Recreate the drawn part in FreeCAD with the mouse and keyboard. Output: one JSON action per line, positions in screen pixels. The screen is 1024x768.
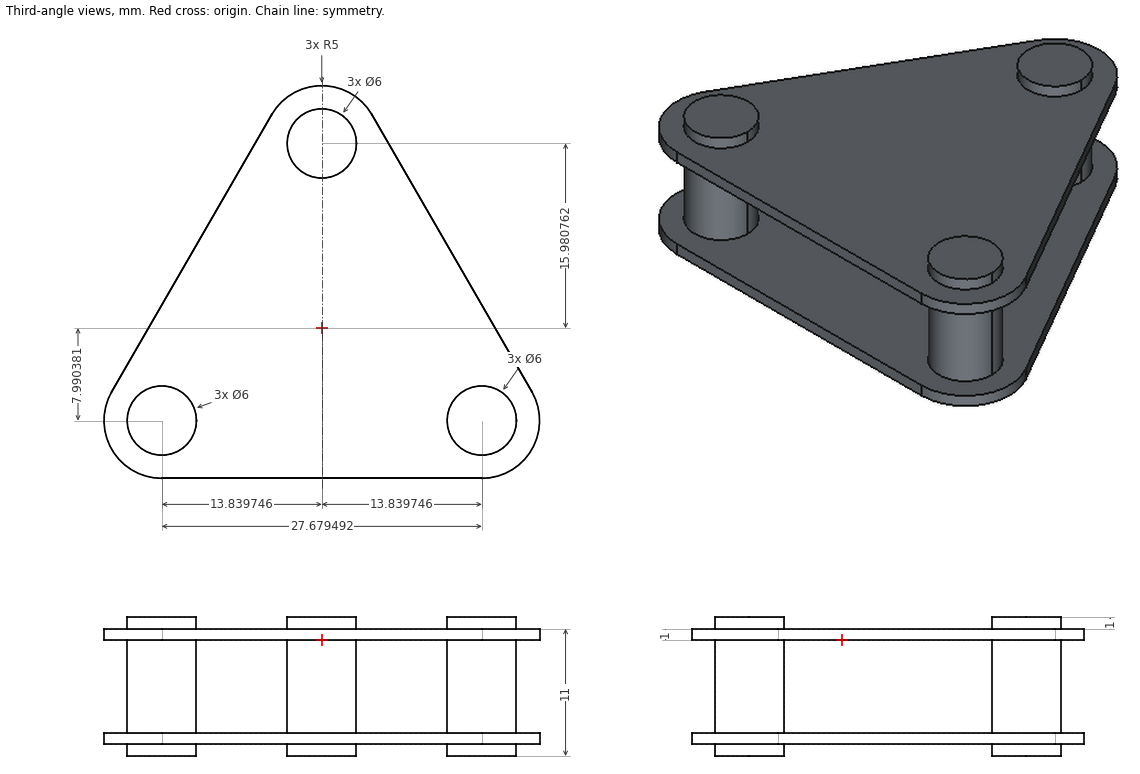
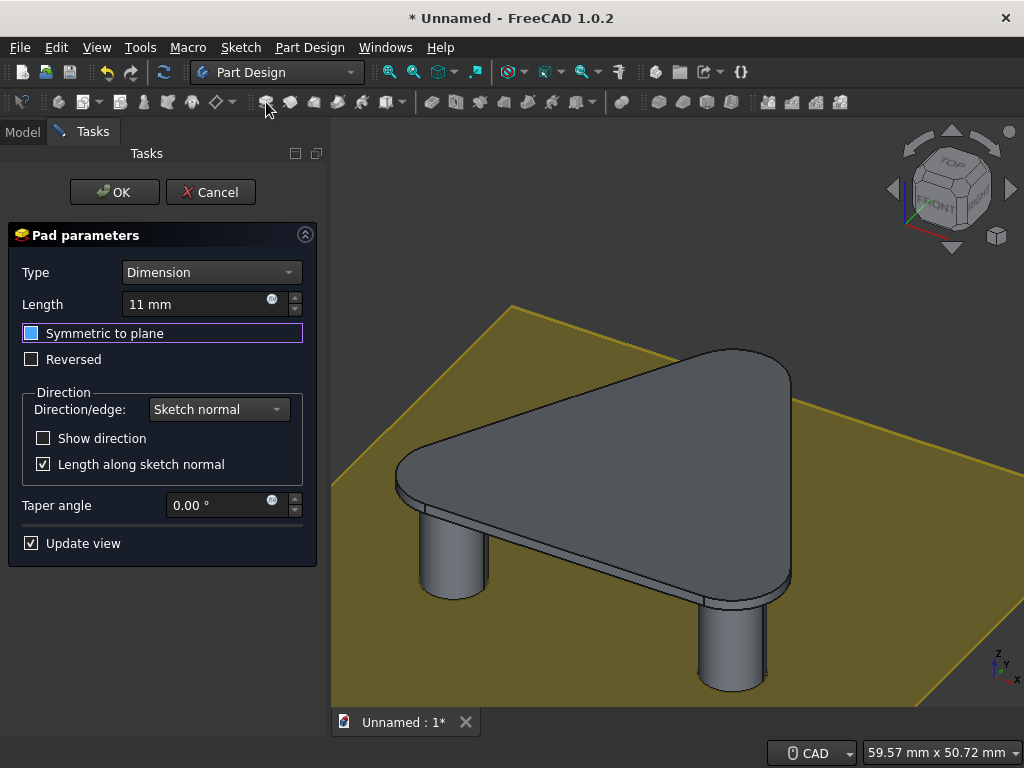
{"action": "left_click", "coordinate": [115, 192]}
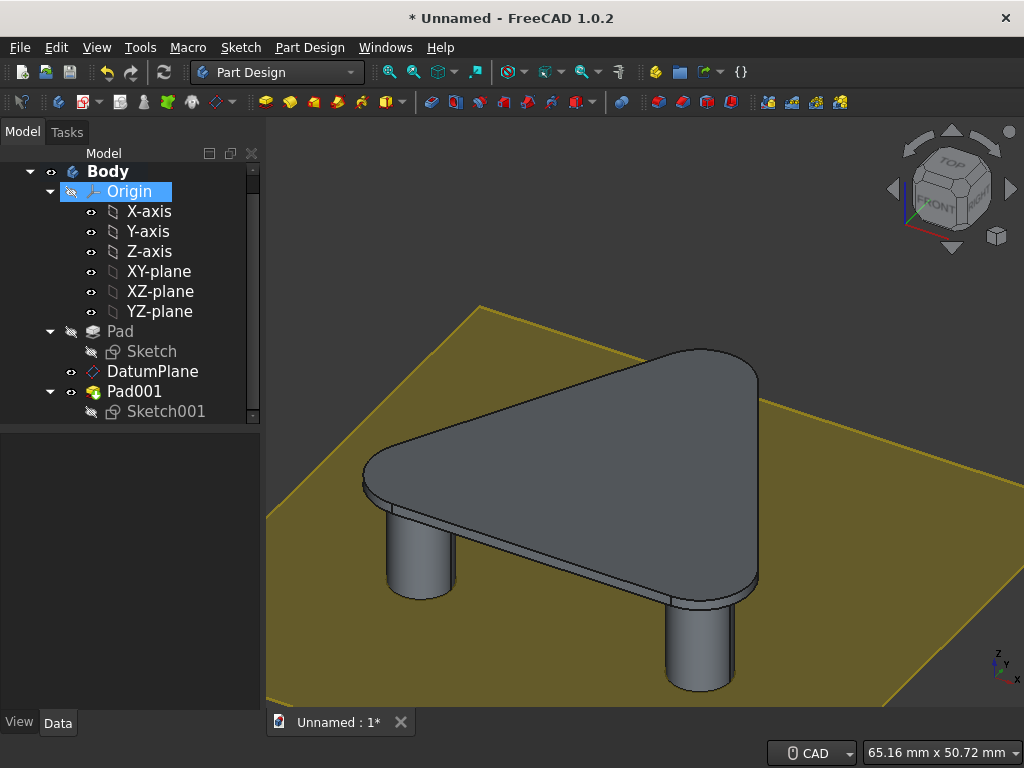
{"action": "left_click", "coordinate": [116, 372]}
{"action": "key", "text": "space"}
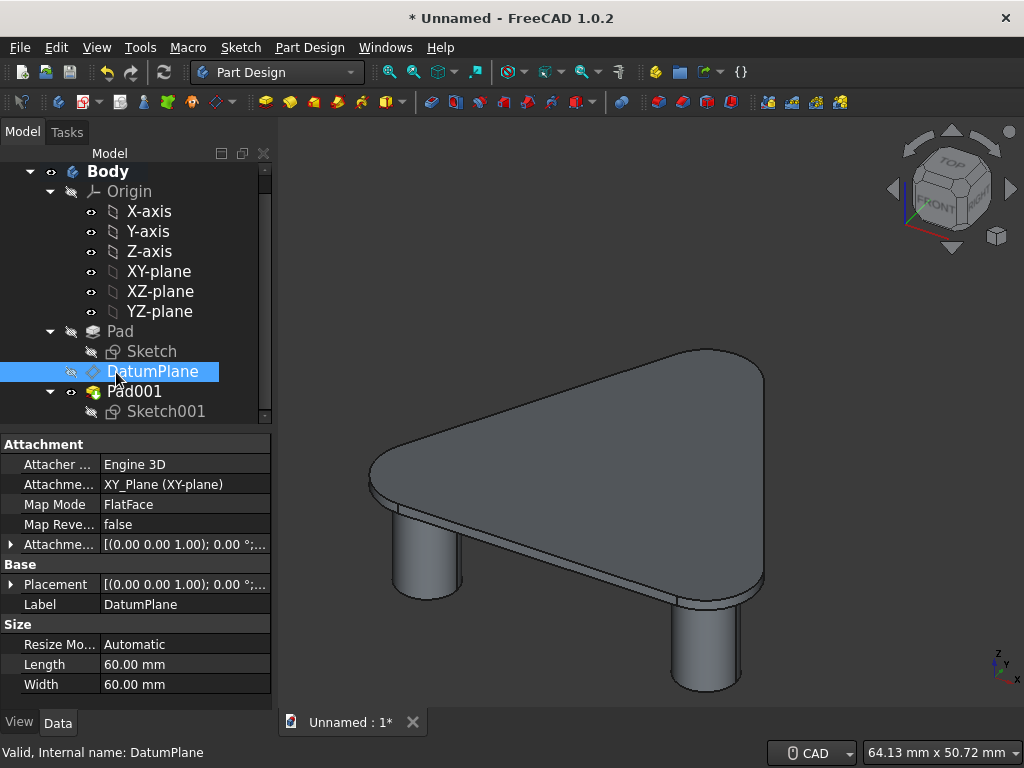
{"action": "left_click", "coordinate": [390, 72]}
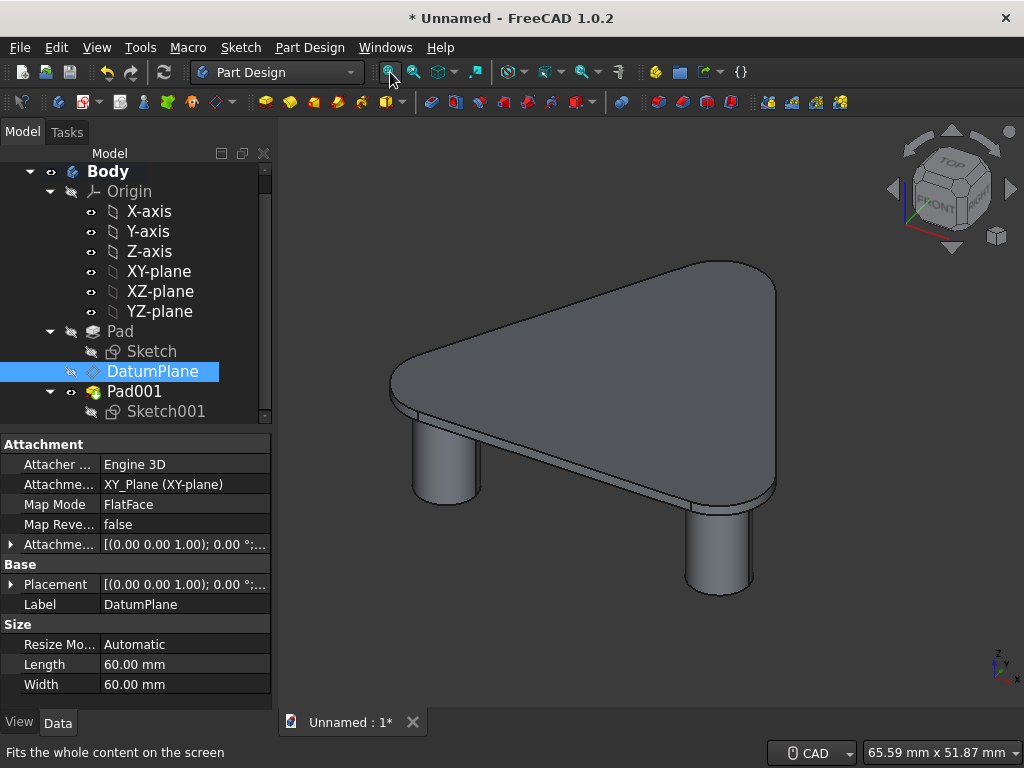
{"action": "left_click", "coordinate": [136, 272]}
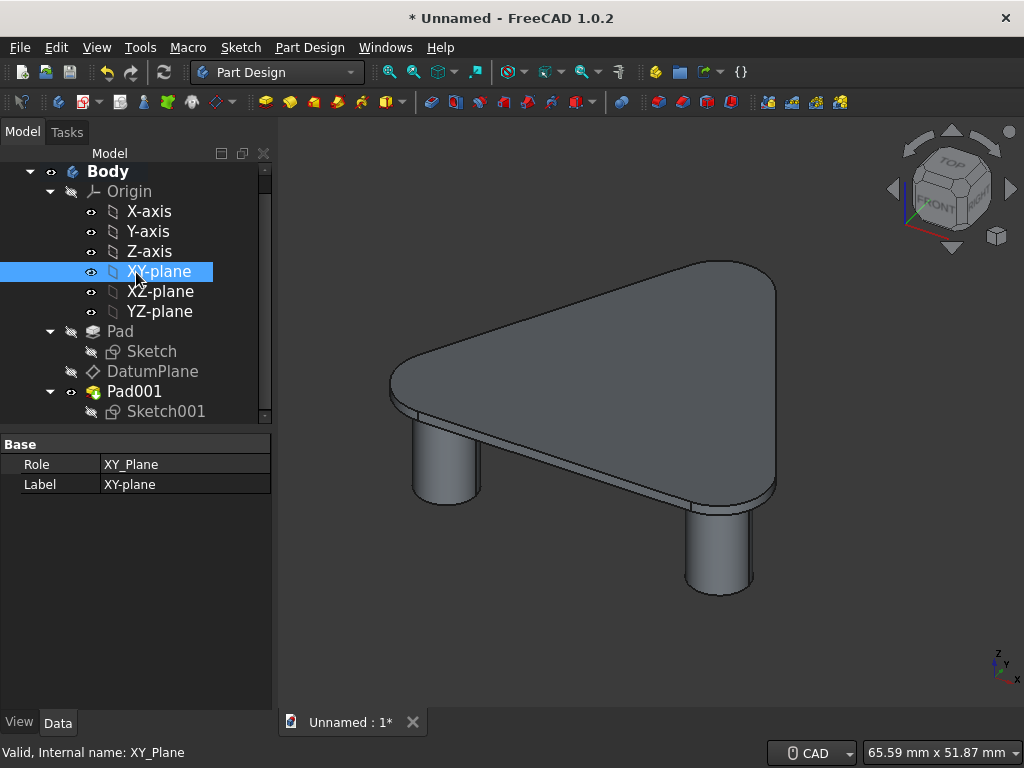
{"action": "left_click", "coordinate": [216, 102]}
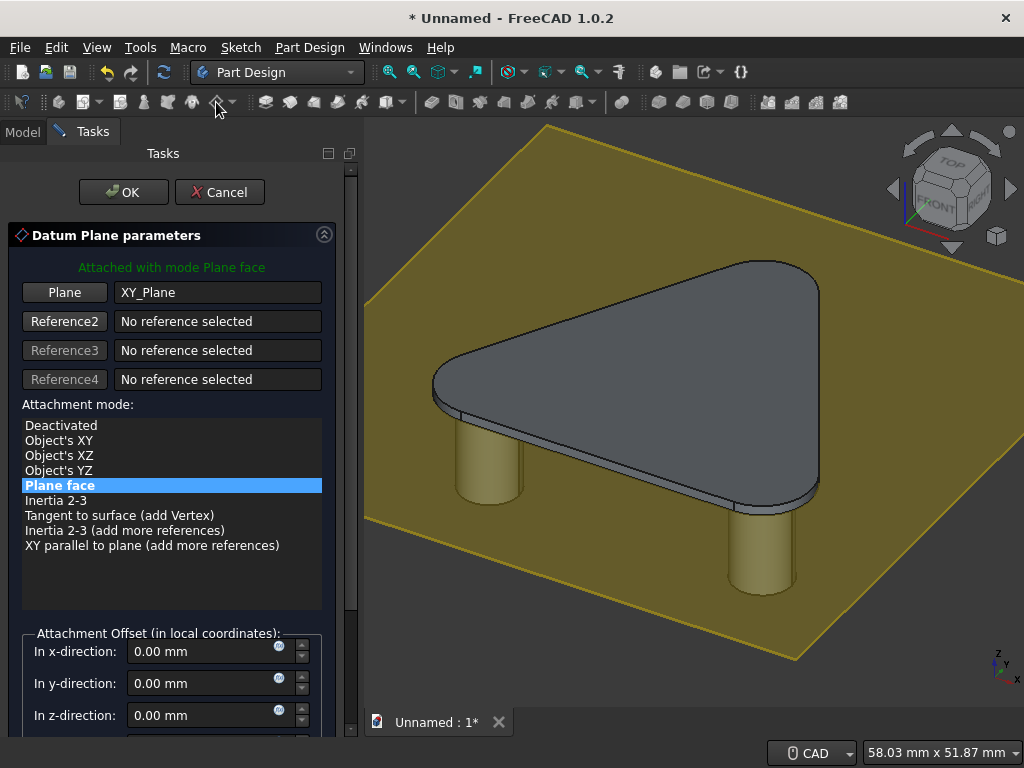
{"action": "triple_click", "coordinate": [210, 715]}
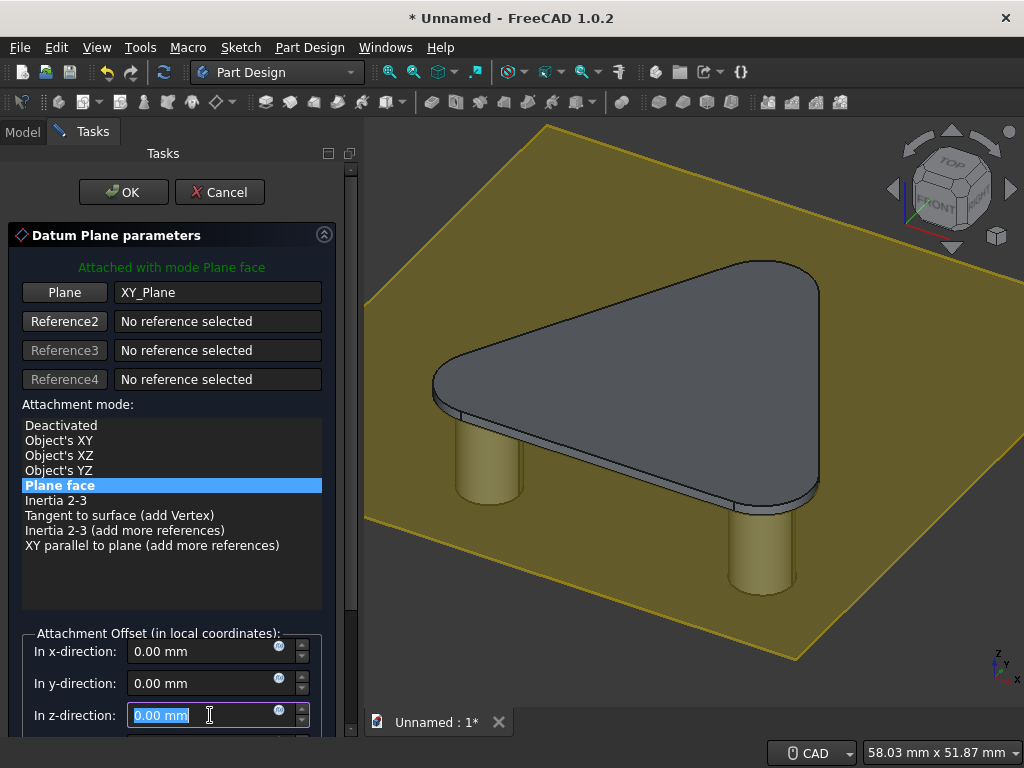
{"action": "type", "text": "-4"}
{"action": "key", "text": "Tab"}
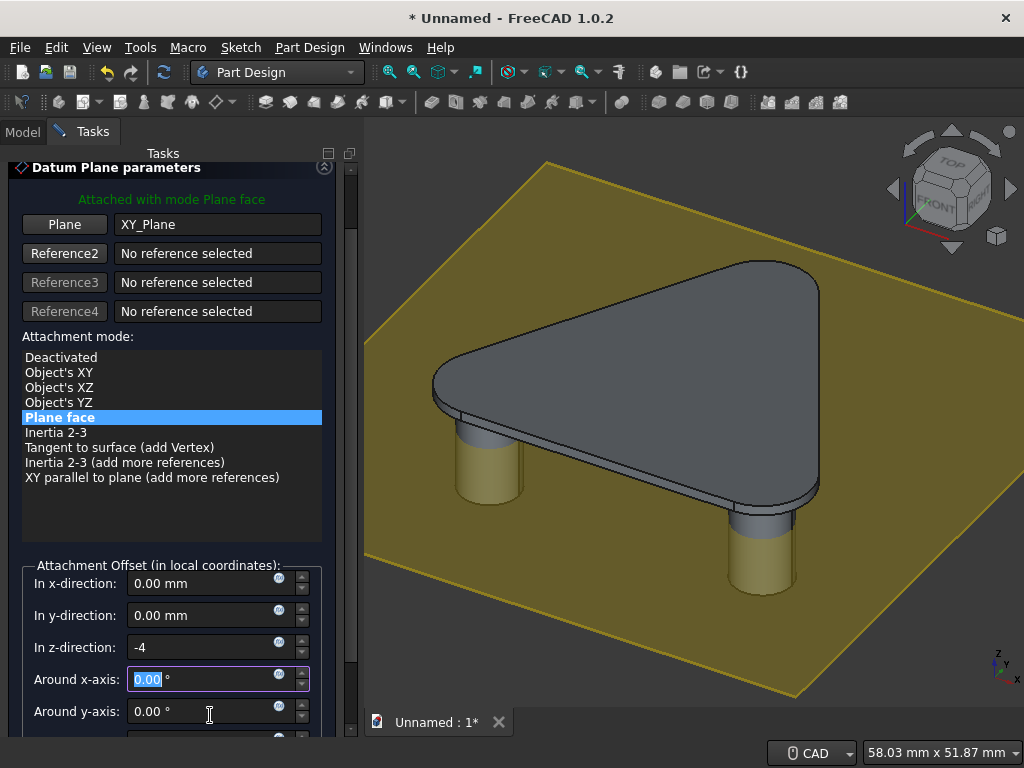
{"action": "scroll", "coordinate": [351, 450], "scroll_direction": "up", "scroll_amount": 2}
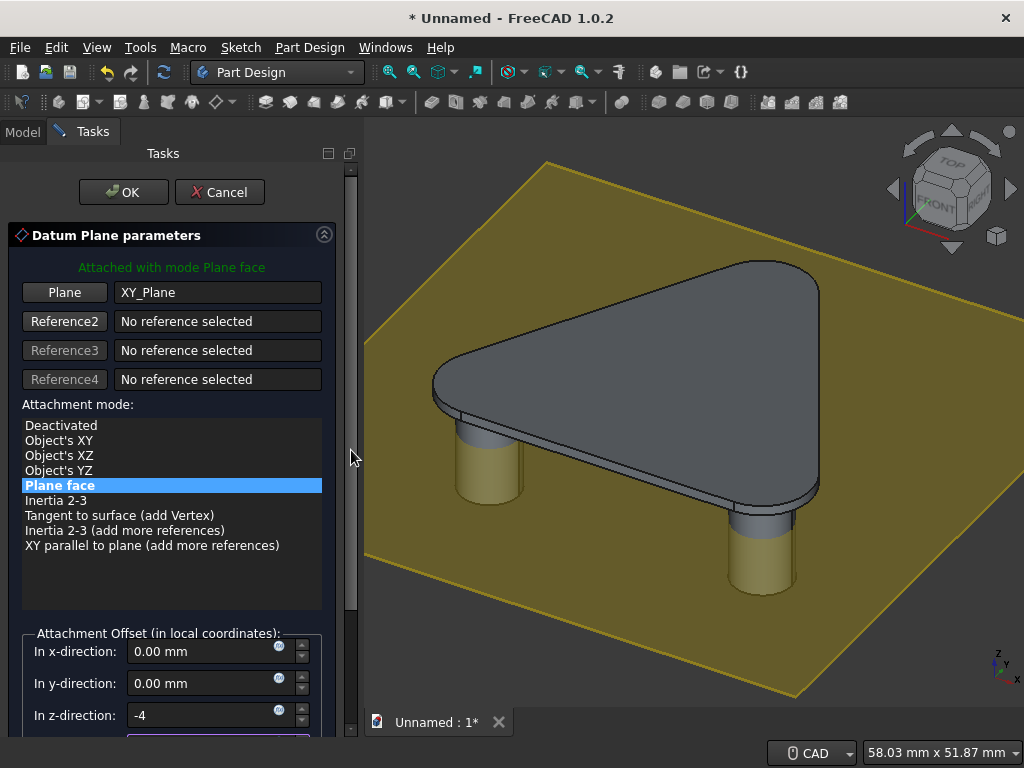
{"action": "left_click", "coordinate": [124, 192]}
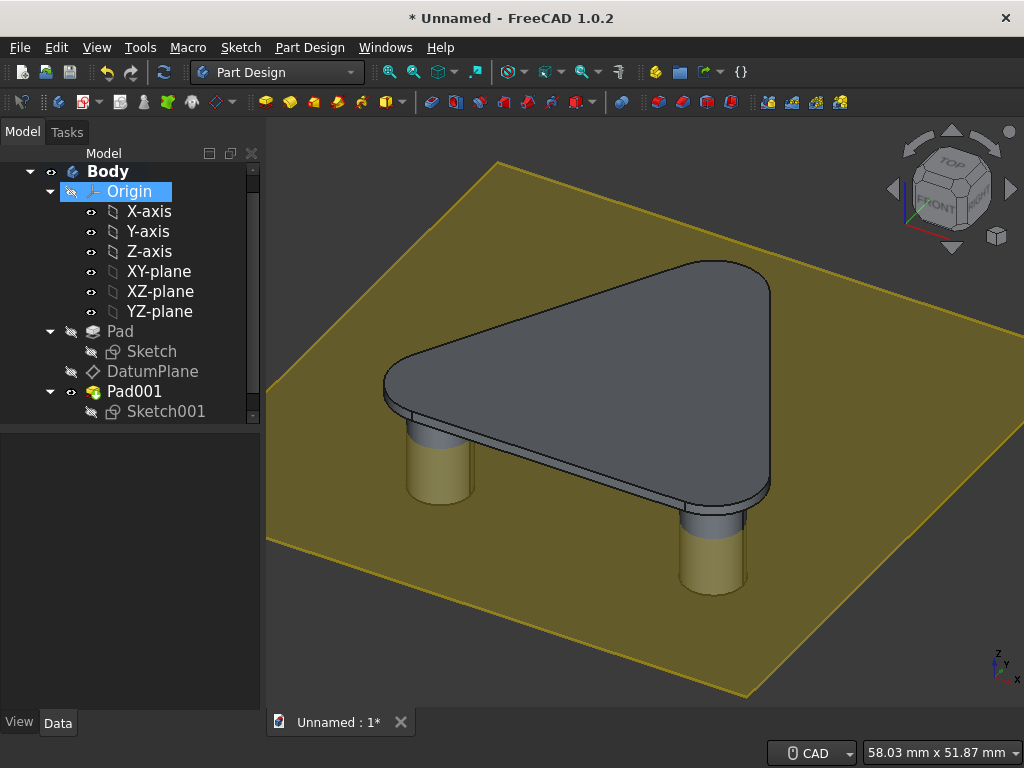
{"action": "left_click", "coordinate": [116, 332]}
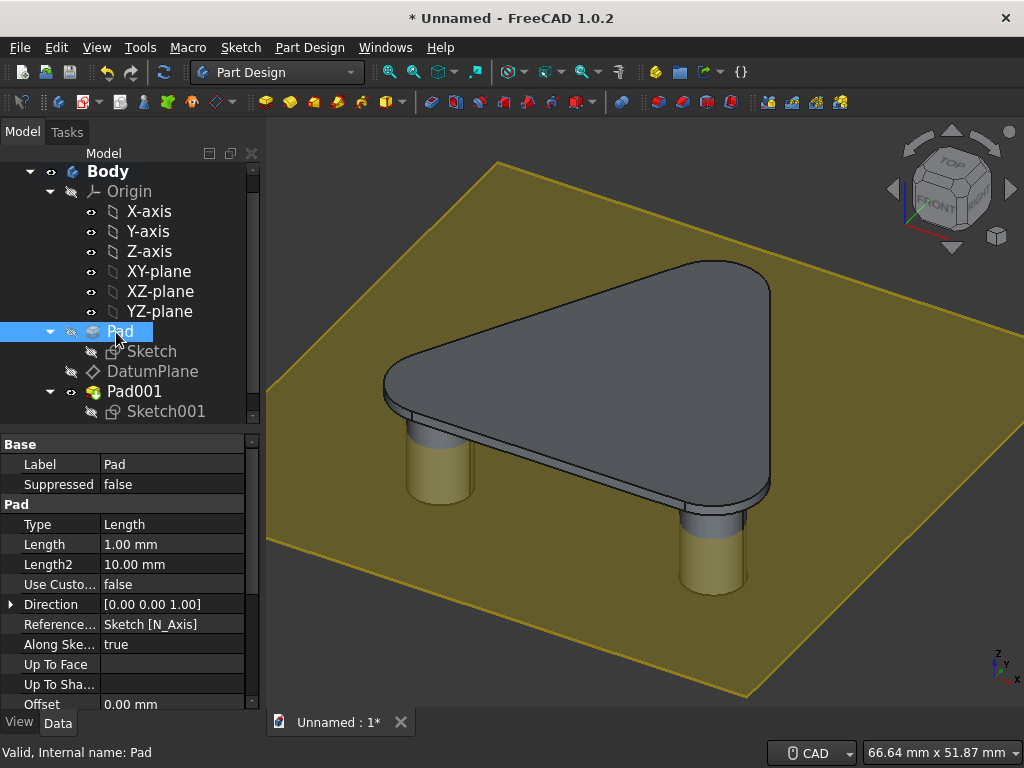
{"action": "left_click", "coordinate": [768, 102]}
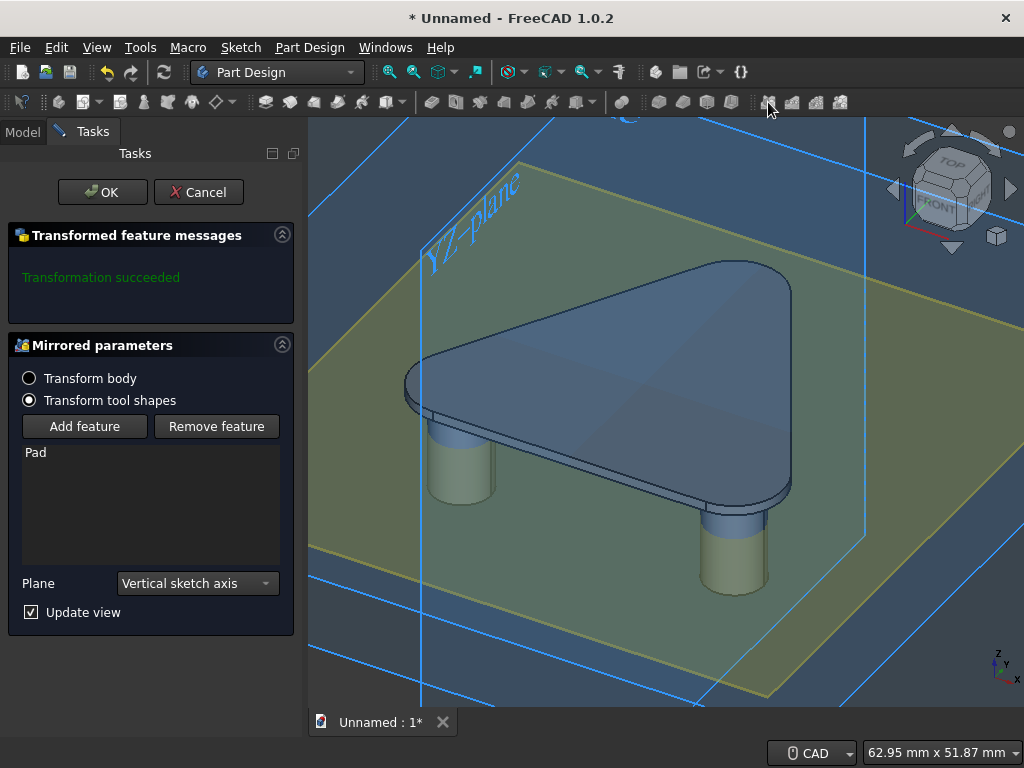
{"action": "left_click", "coordinate": [198, 584]}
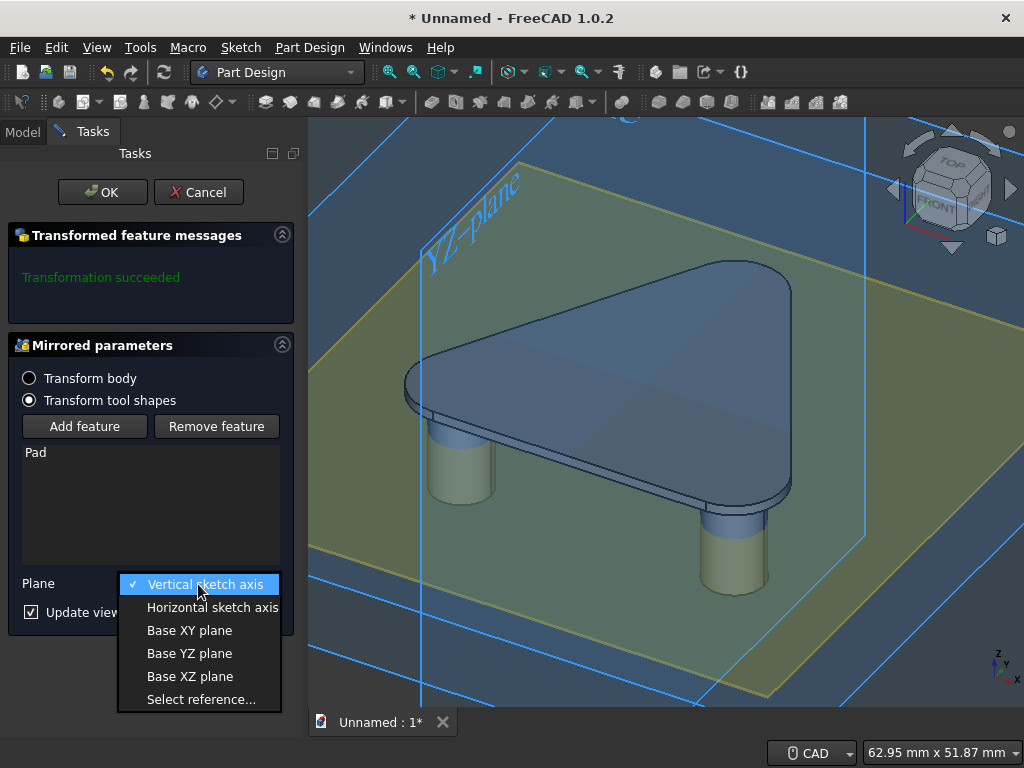
{"action": "left_click", "coordinate": [198, 700]}